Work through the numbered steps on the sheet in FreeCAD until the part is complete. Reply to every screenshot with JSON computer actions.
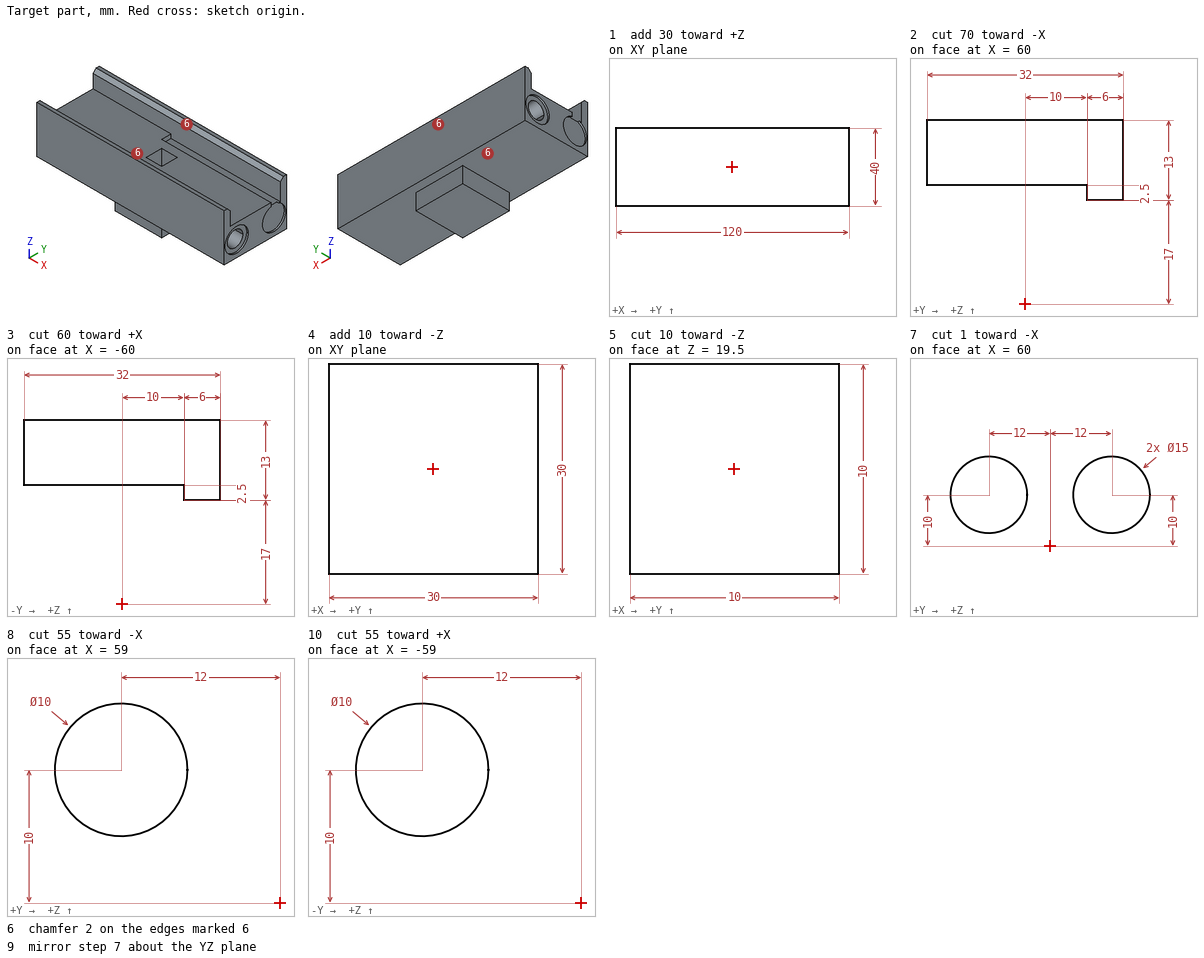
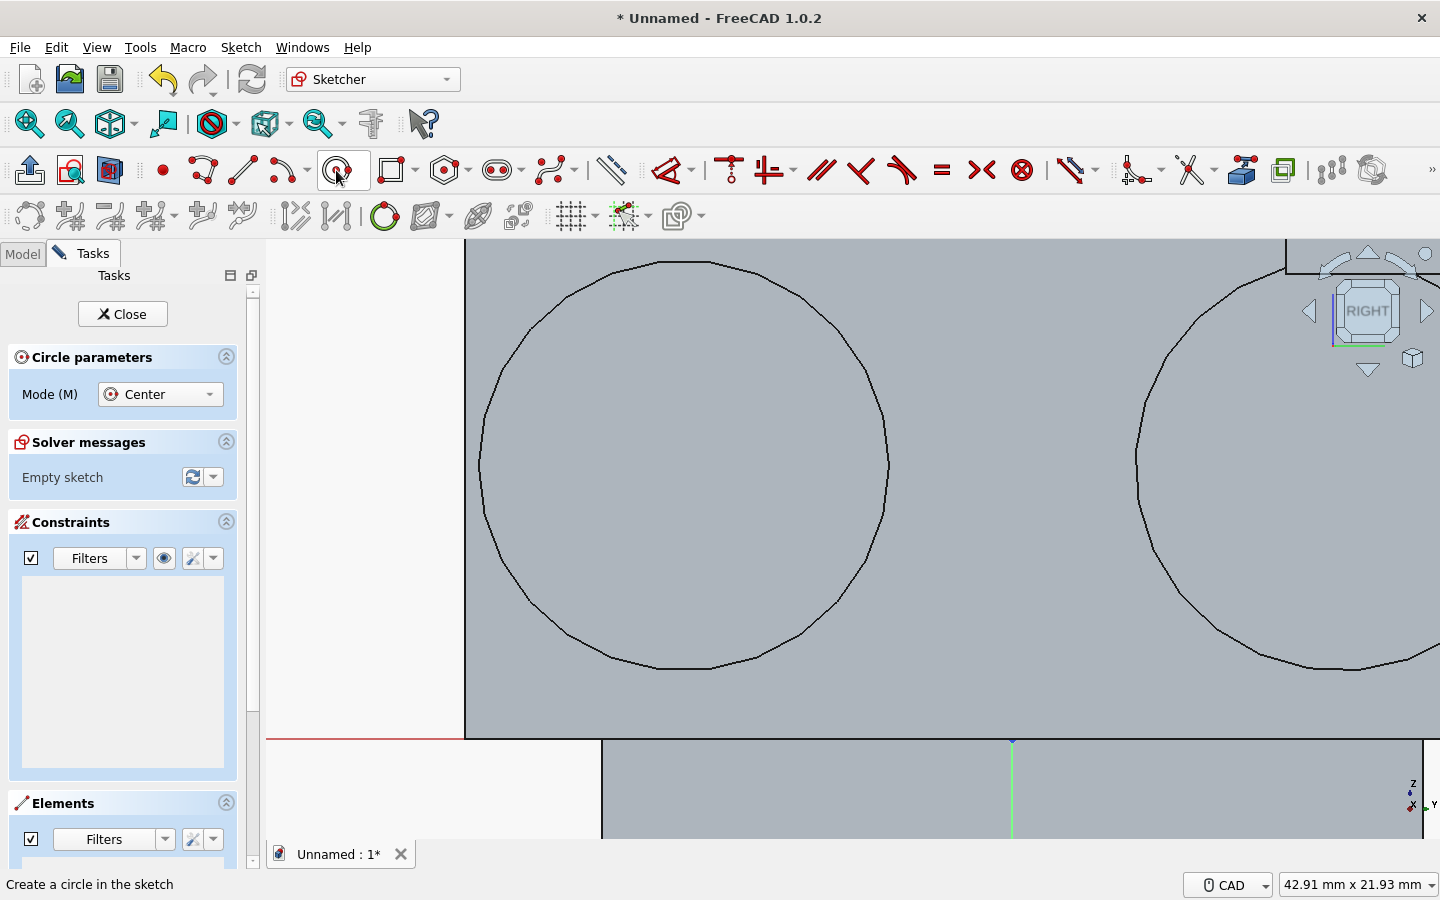
{"action": "left_click", "coordinate": [684, 466]}
{"action": "mouse_move", "coordinate": [781, 369]}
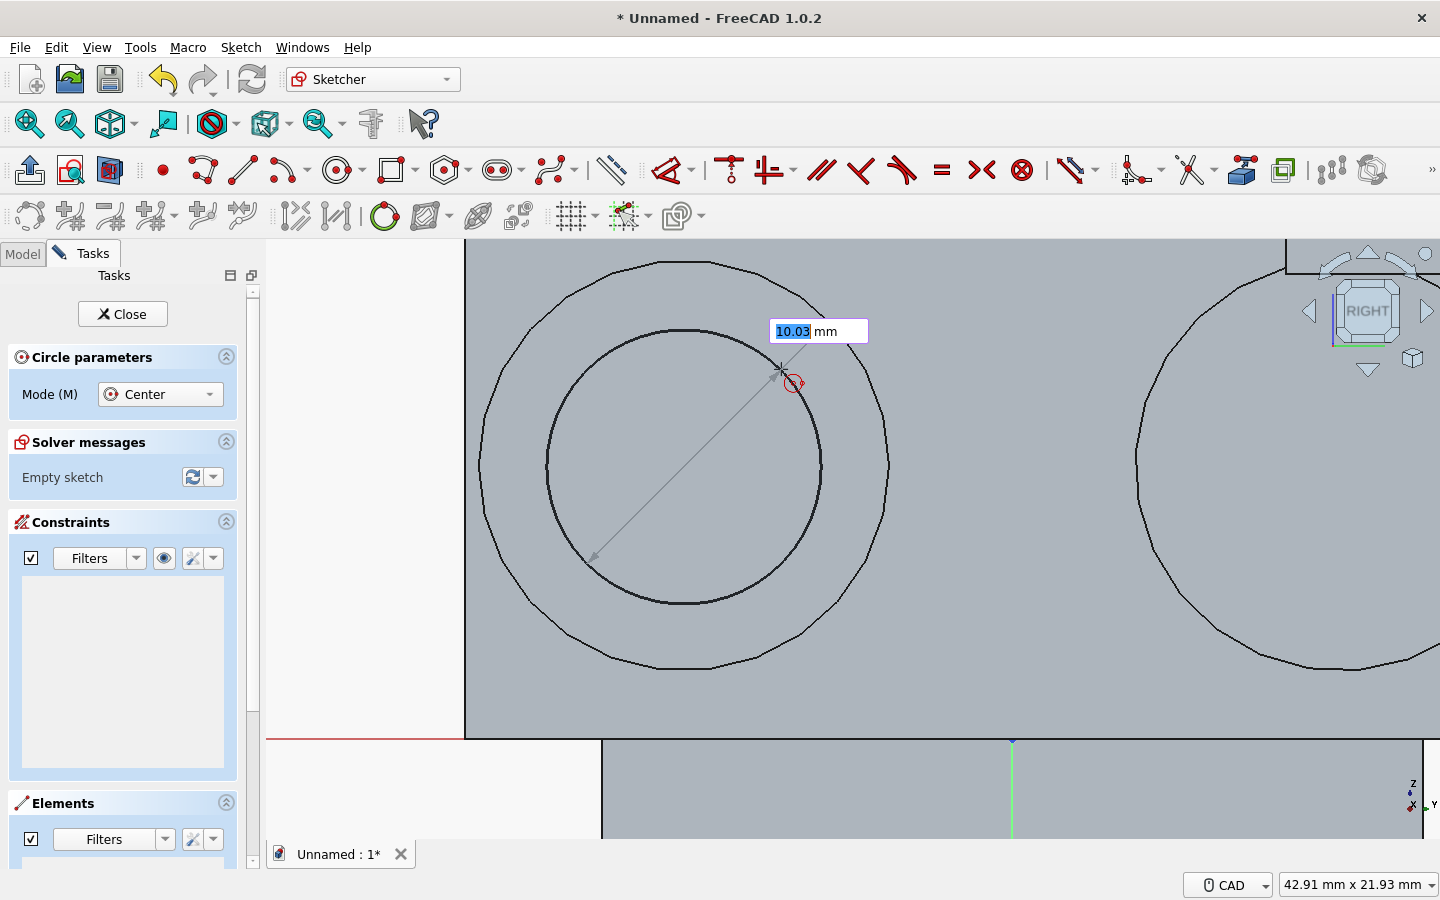
{"action": "type", "text": "10"}
{"action": "key", "text": "Return"}
{"action": "key", "text": "Escape"}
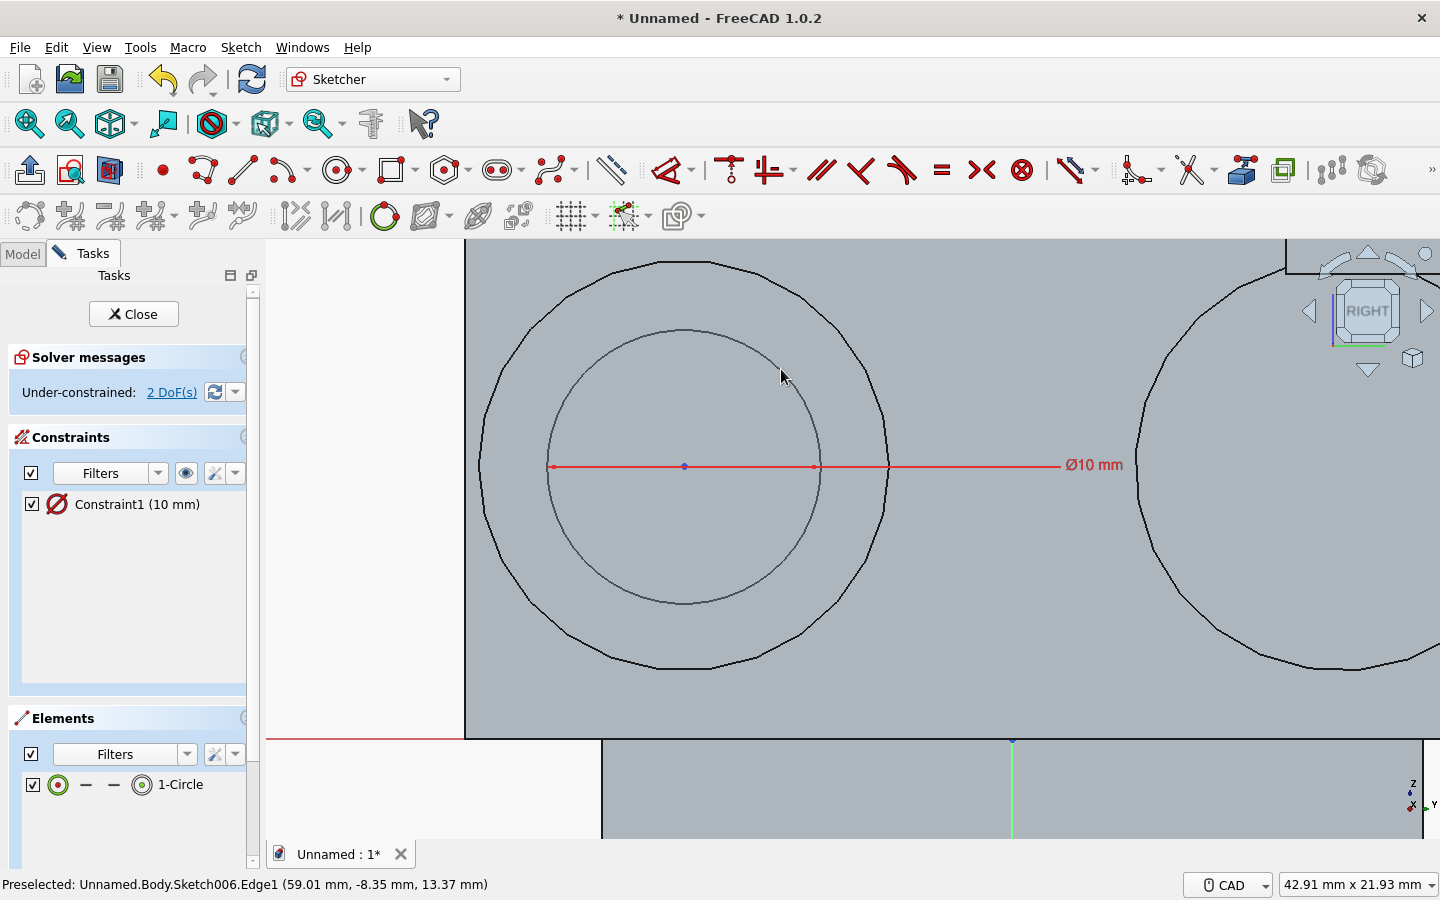
{"action": "key", "text": "d"}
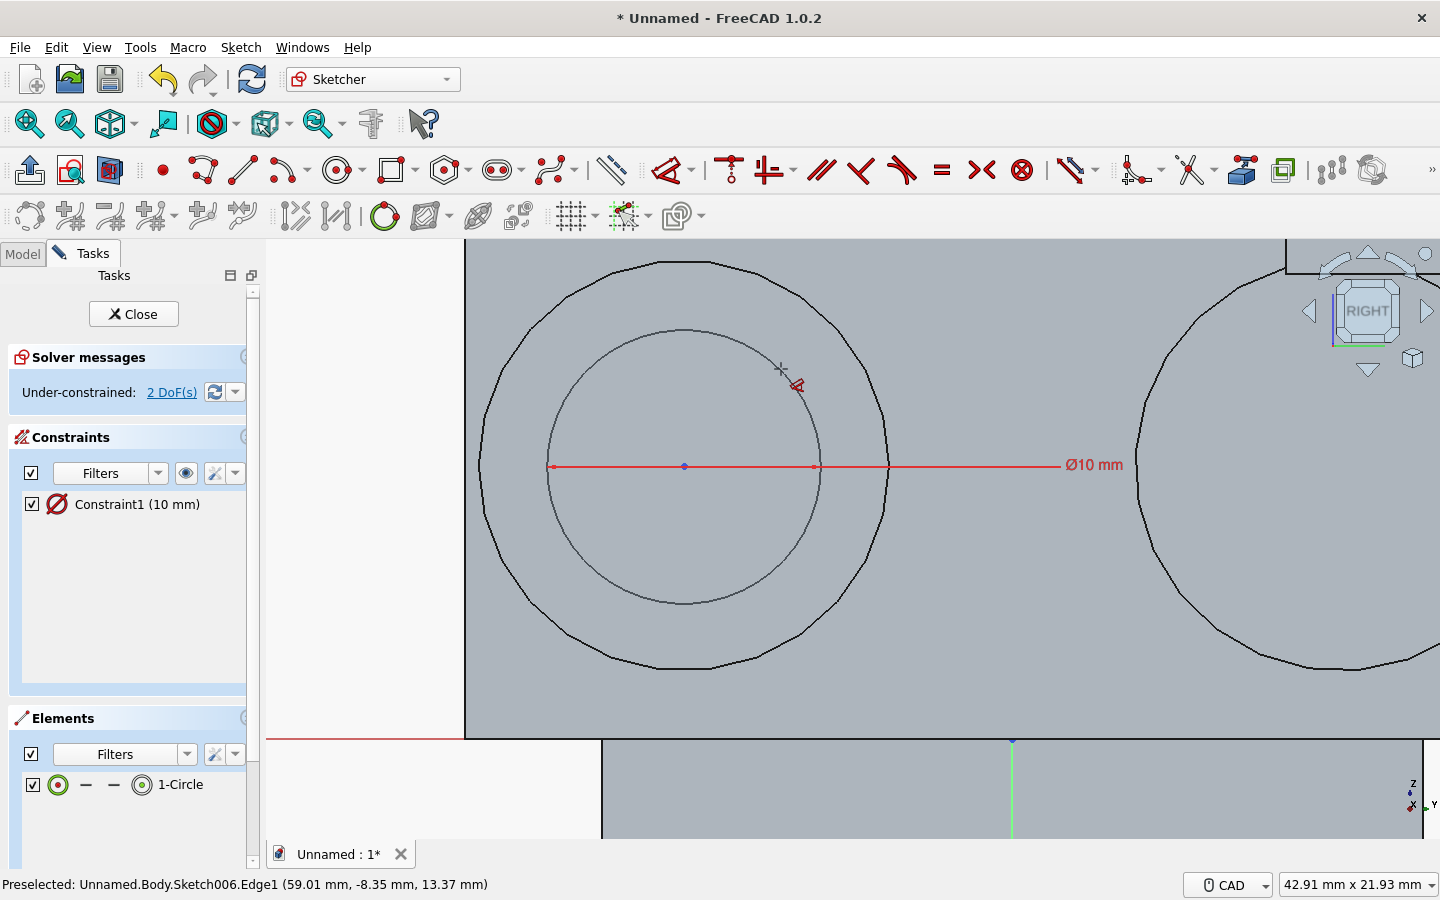
{"action": "left_click", "coordinate": [684, 467]}
{"action": "left_click", "coordinate": [848, 773]}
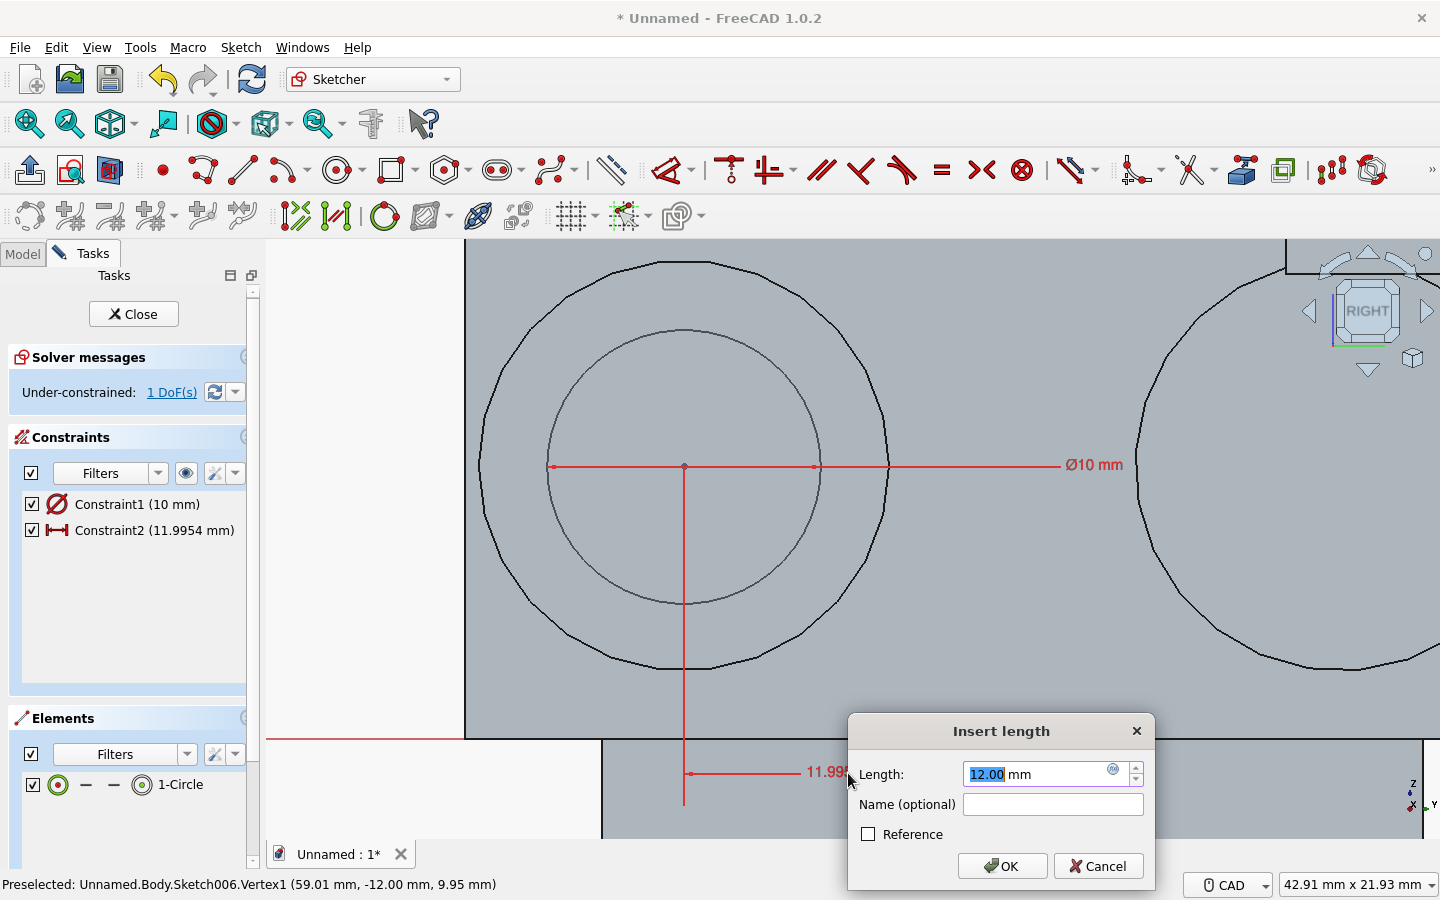
{"action": "type", "text": "12"}
{"action": "key", "text": "Return"}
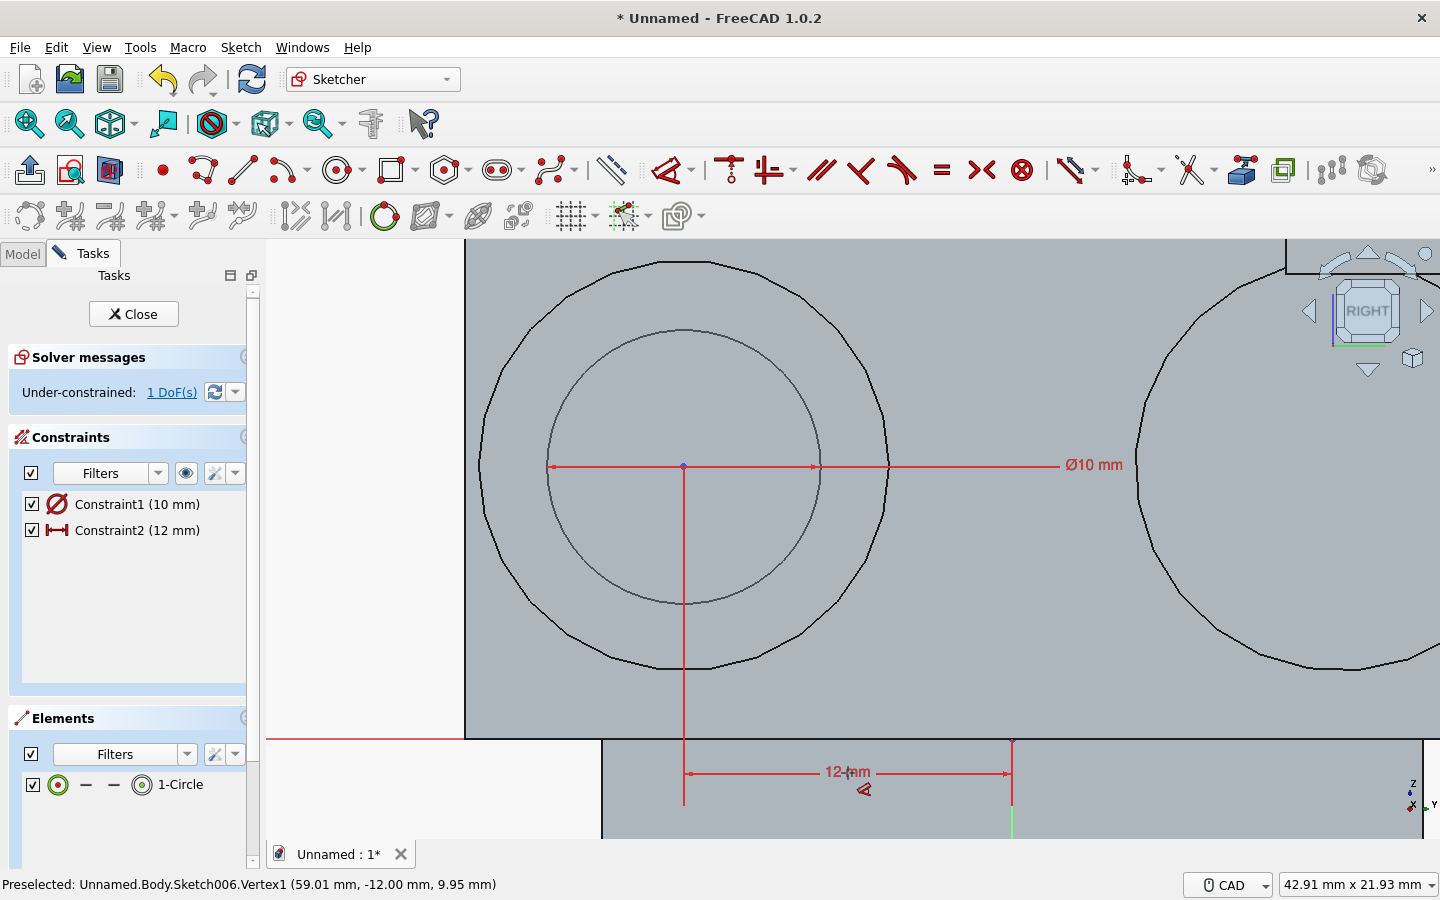
{"action": "left_click", "coordinate": [684, 467]}
{"action": "left_click", "coordinate": [1046, 603]}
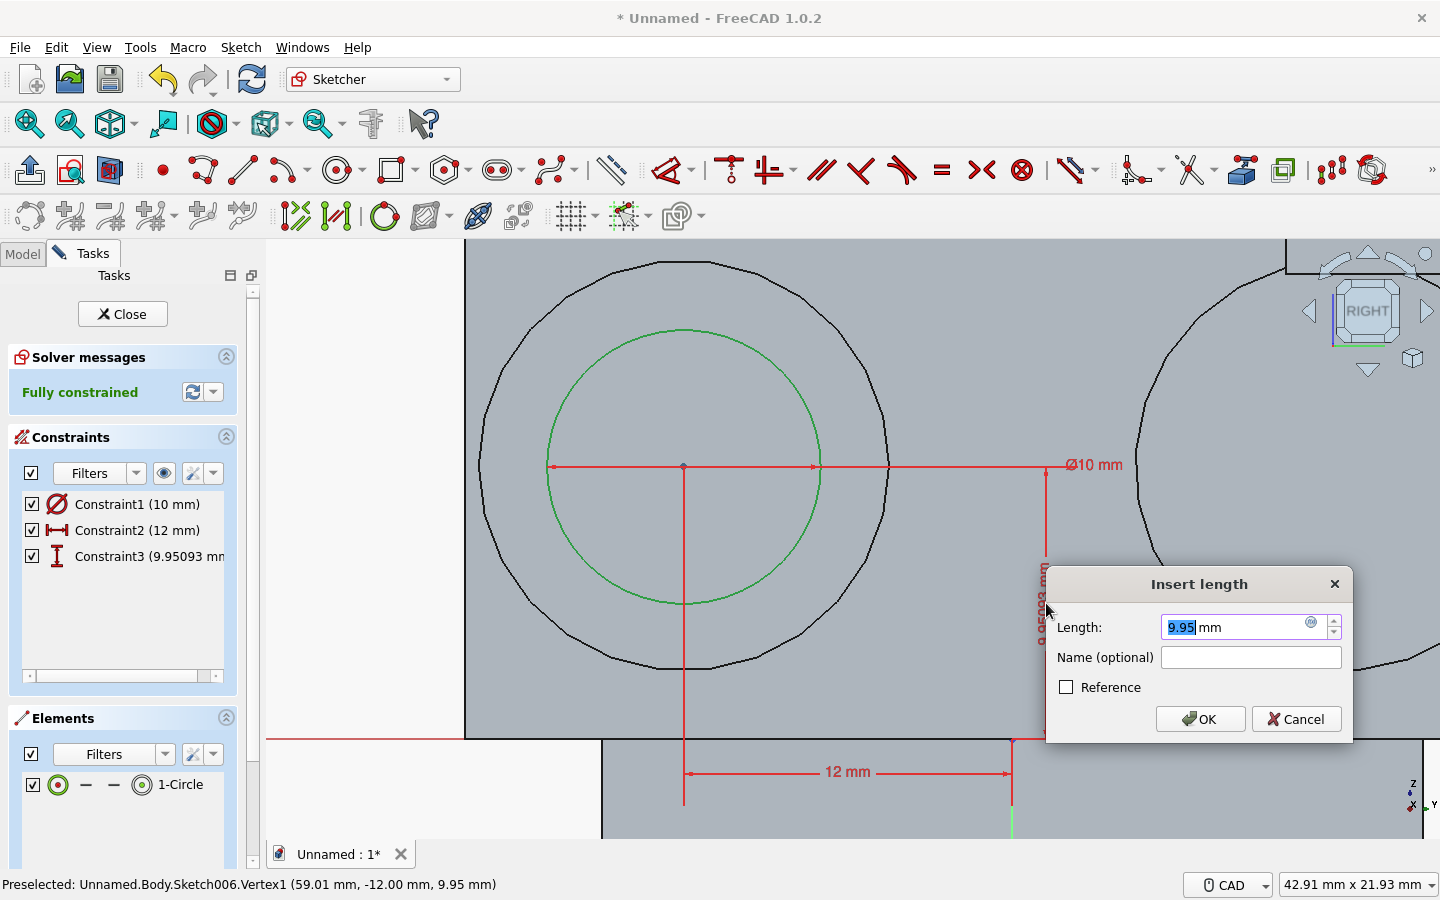
{"action": "type", "text": "10"}
{"action": "key", "text": "Return"}
{"action": "key", "text": "Escape"}